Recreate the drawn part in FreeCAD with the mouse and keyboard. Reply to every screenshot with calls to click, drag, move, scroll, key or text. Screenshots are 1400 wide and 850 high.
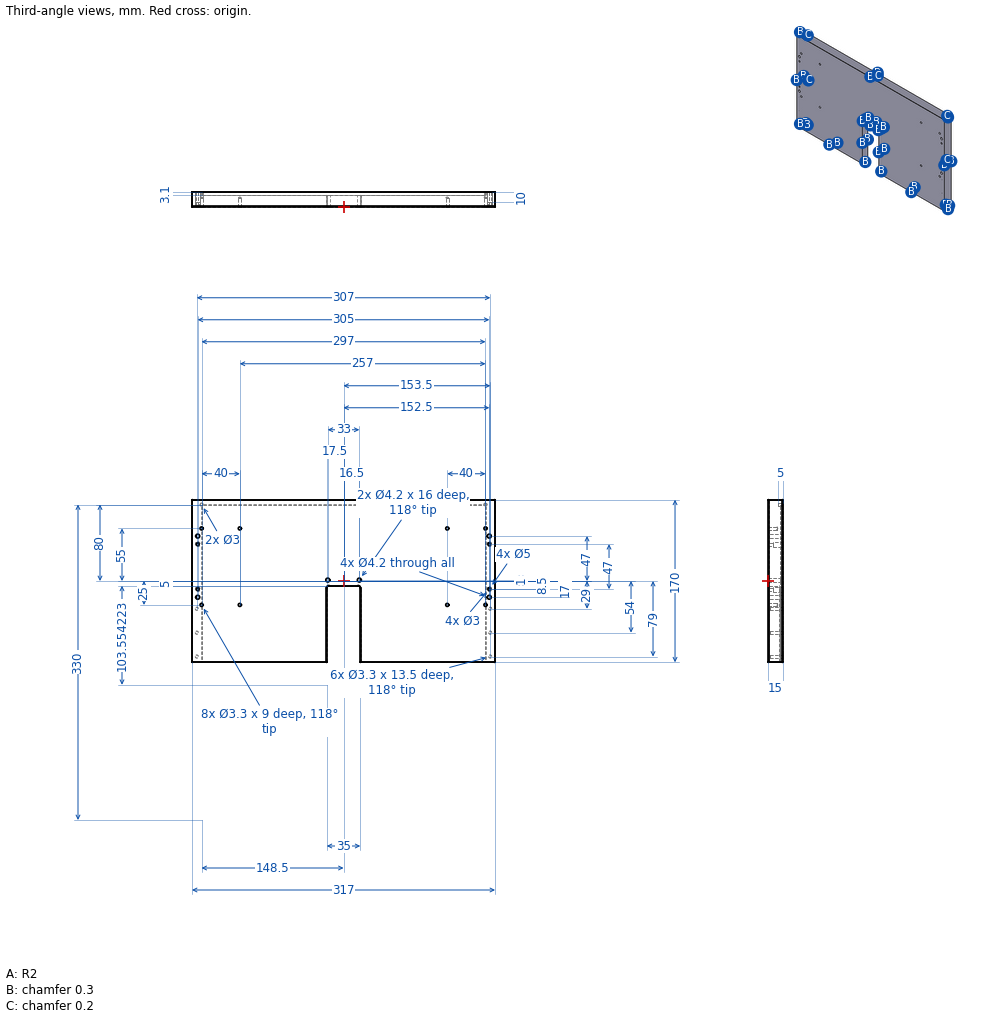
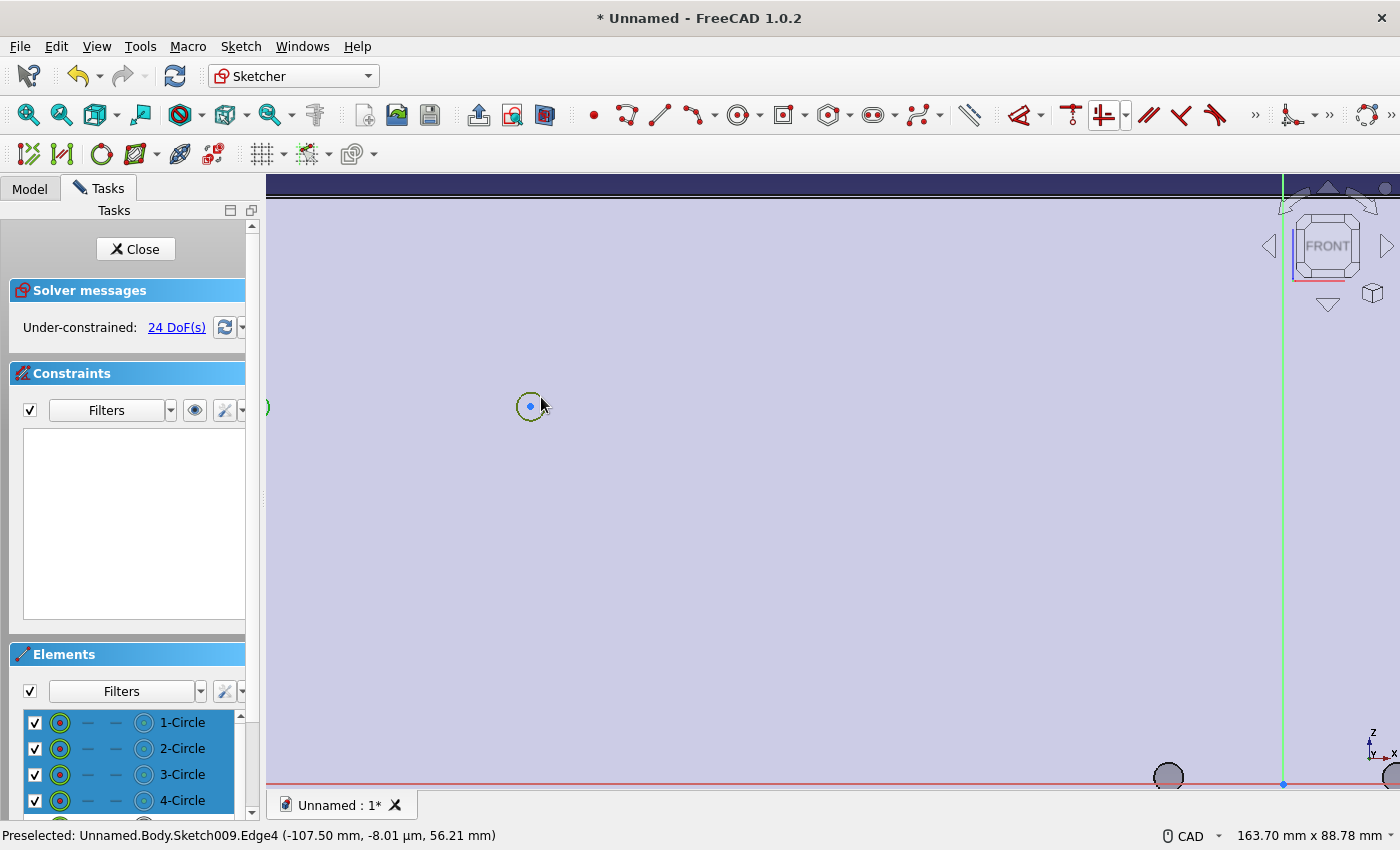
scroll(541, 396, down, 6)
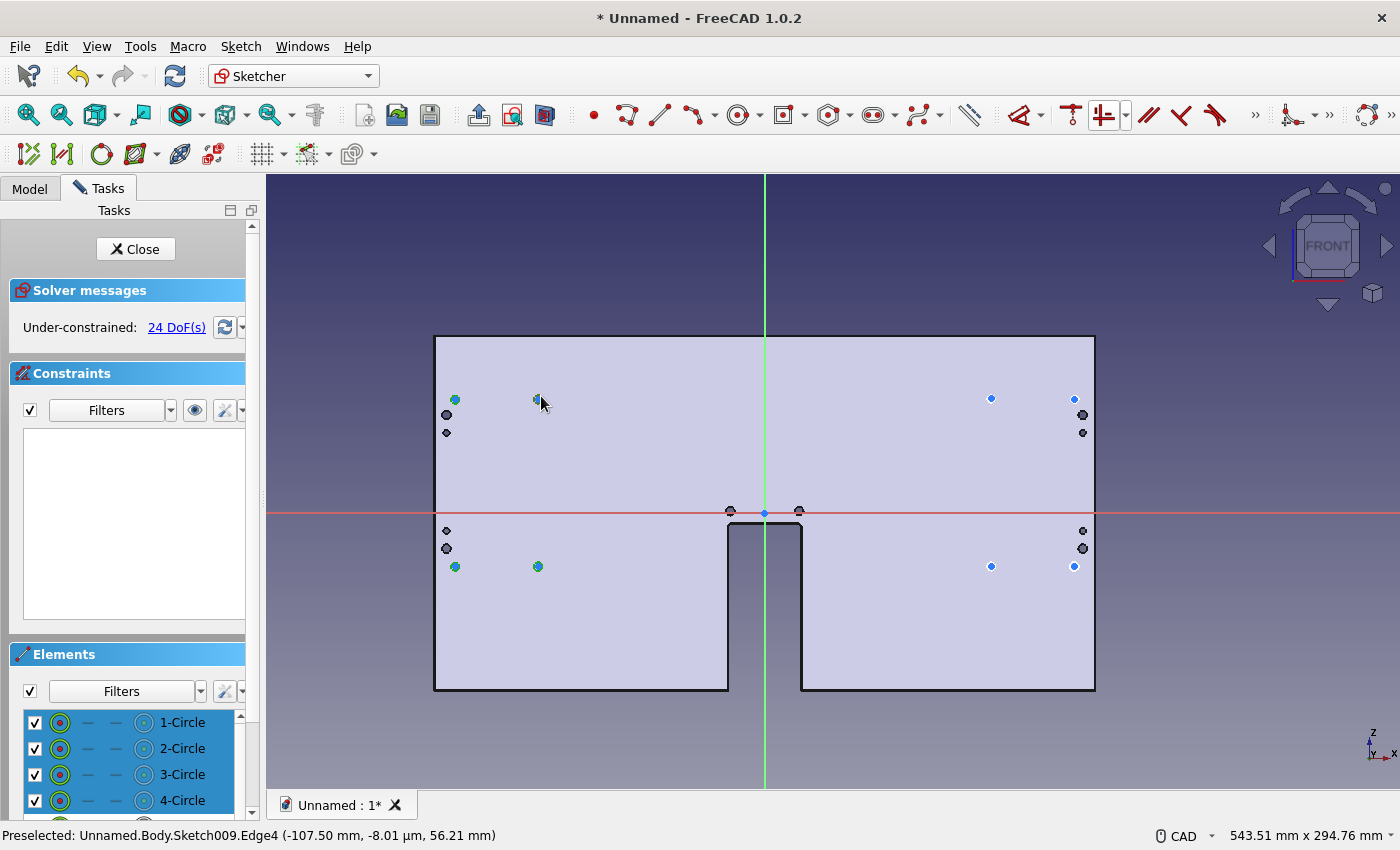
scroll(1077, 563, up, 6)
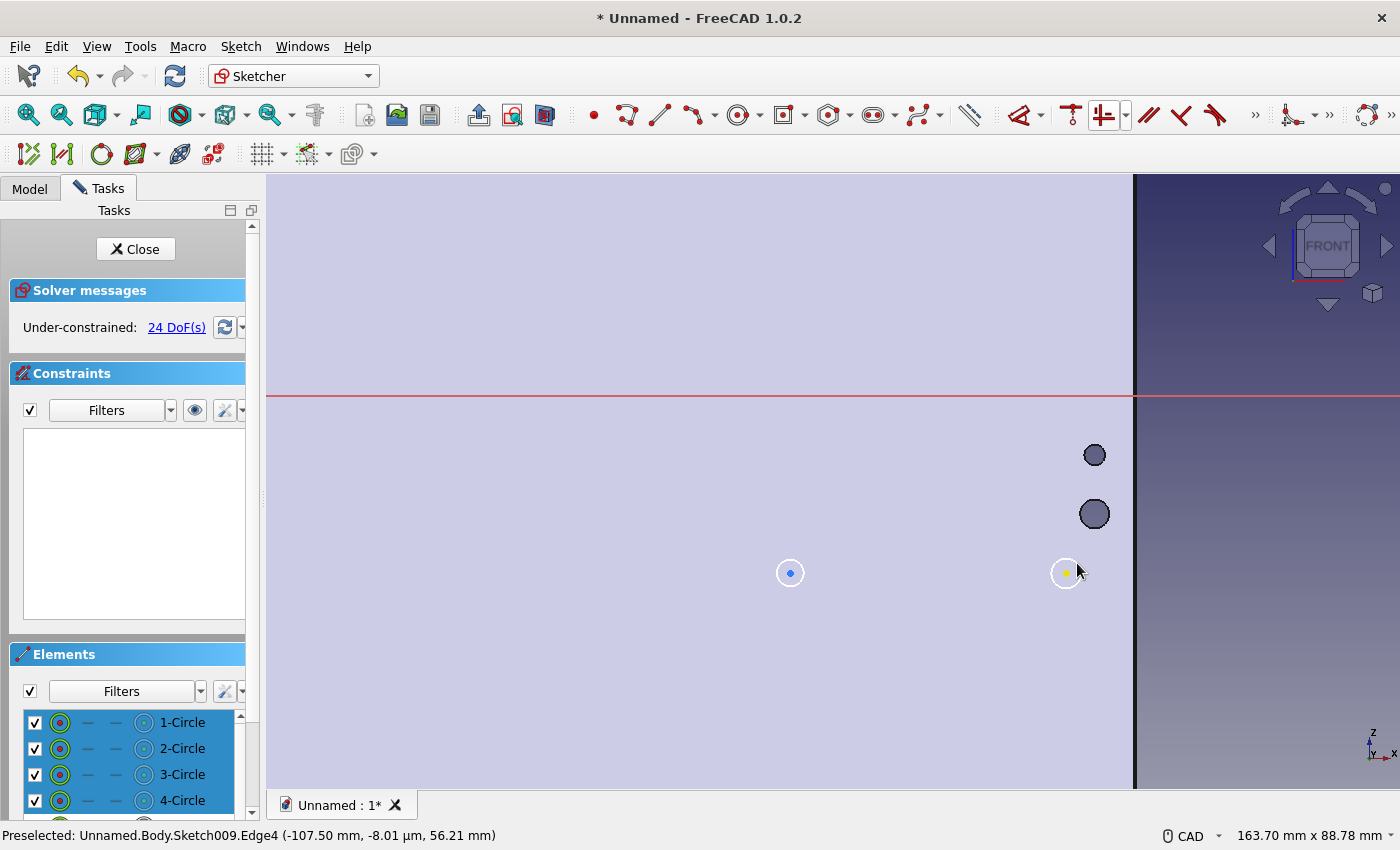
click(1077, 563)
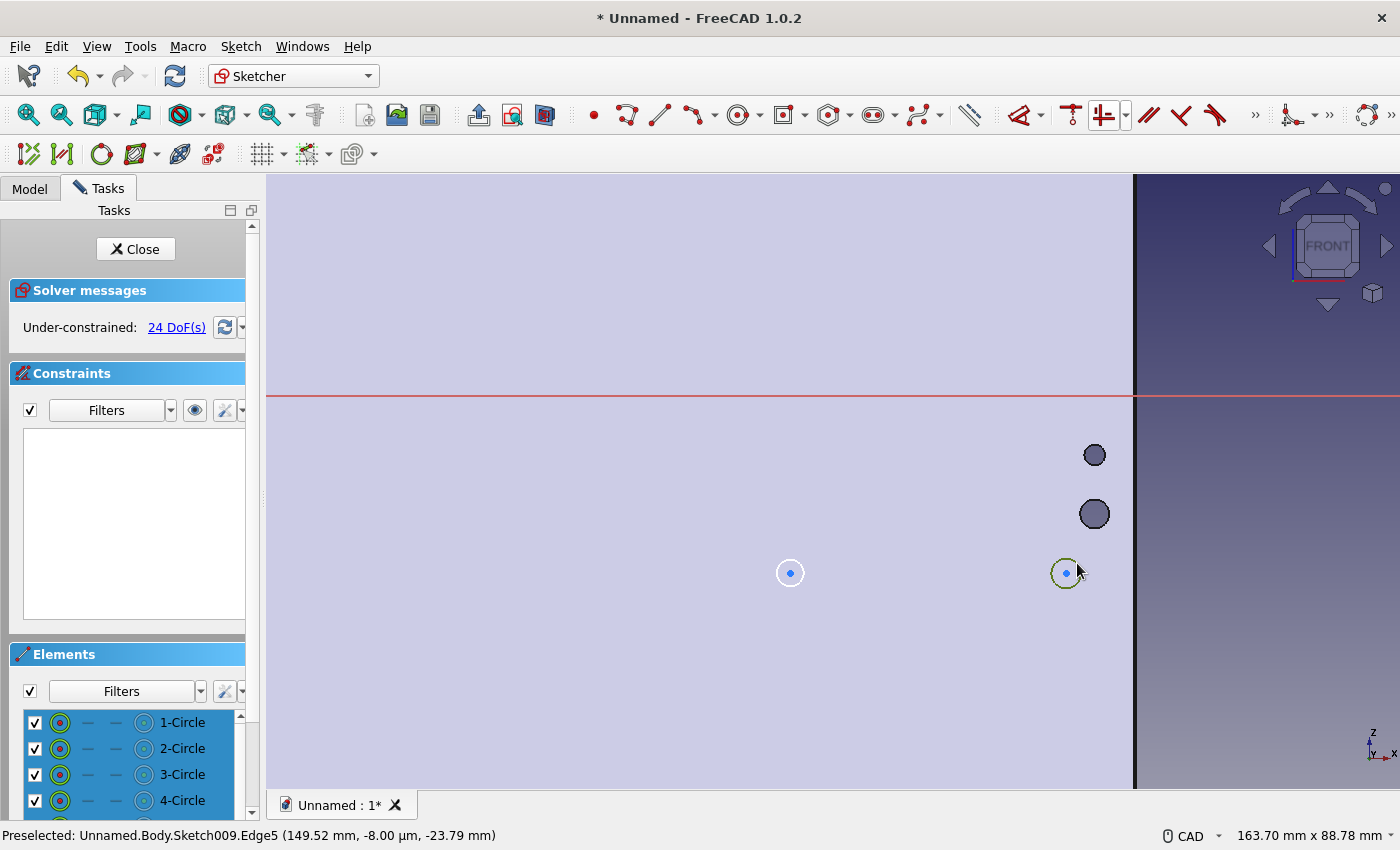
click(800, 564)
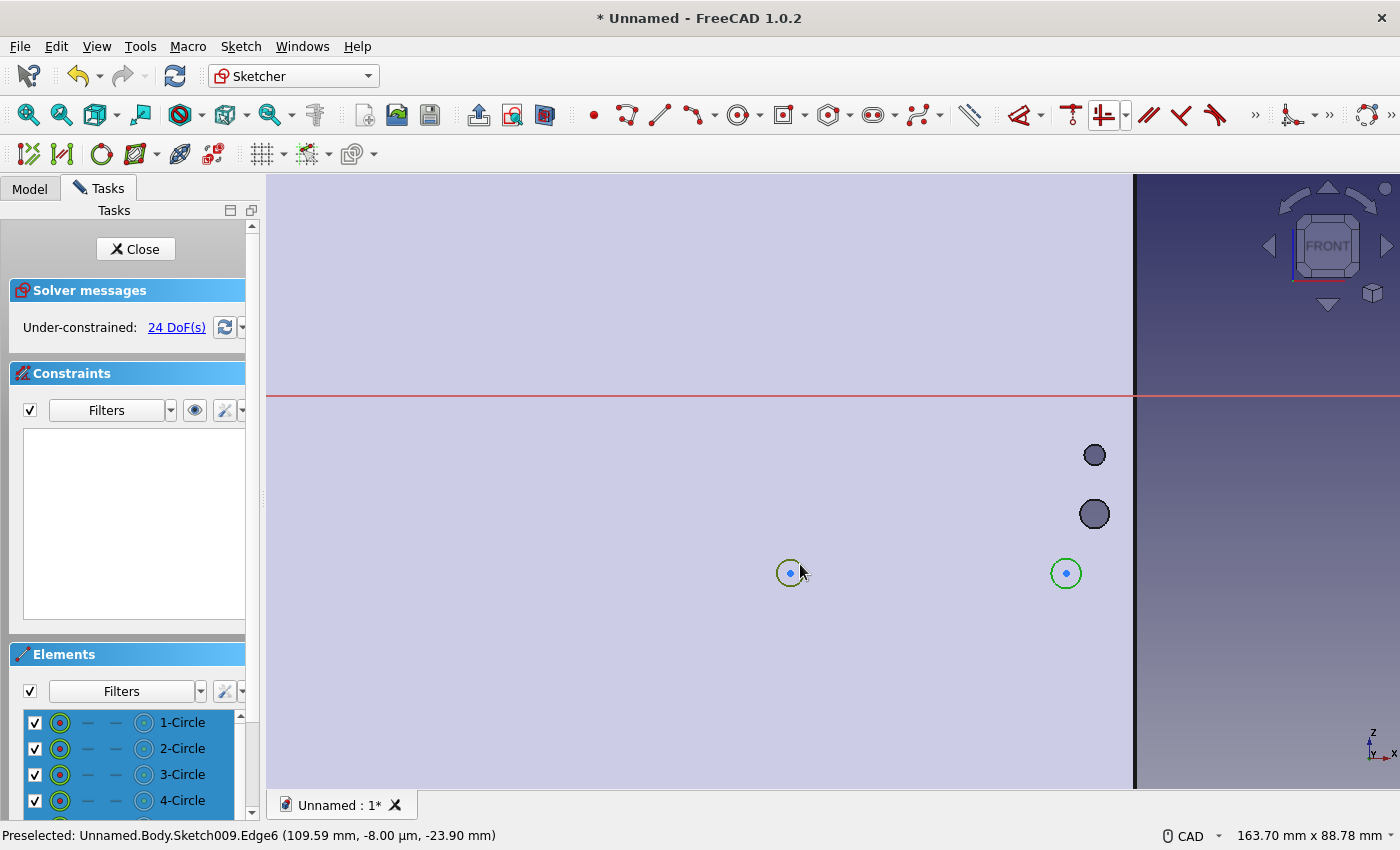
scroll(1077, 563, down, 6)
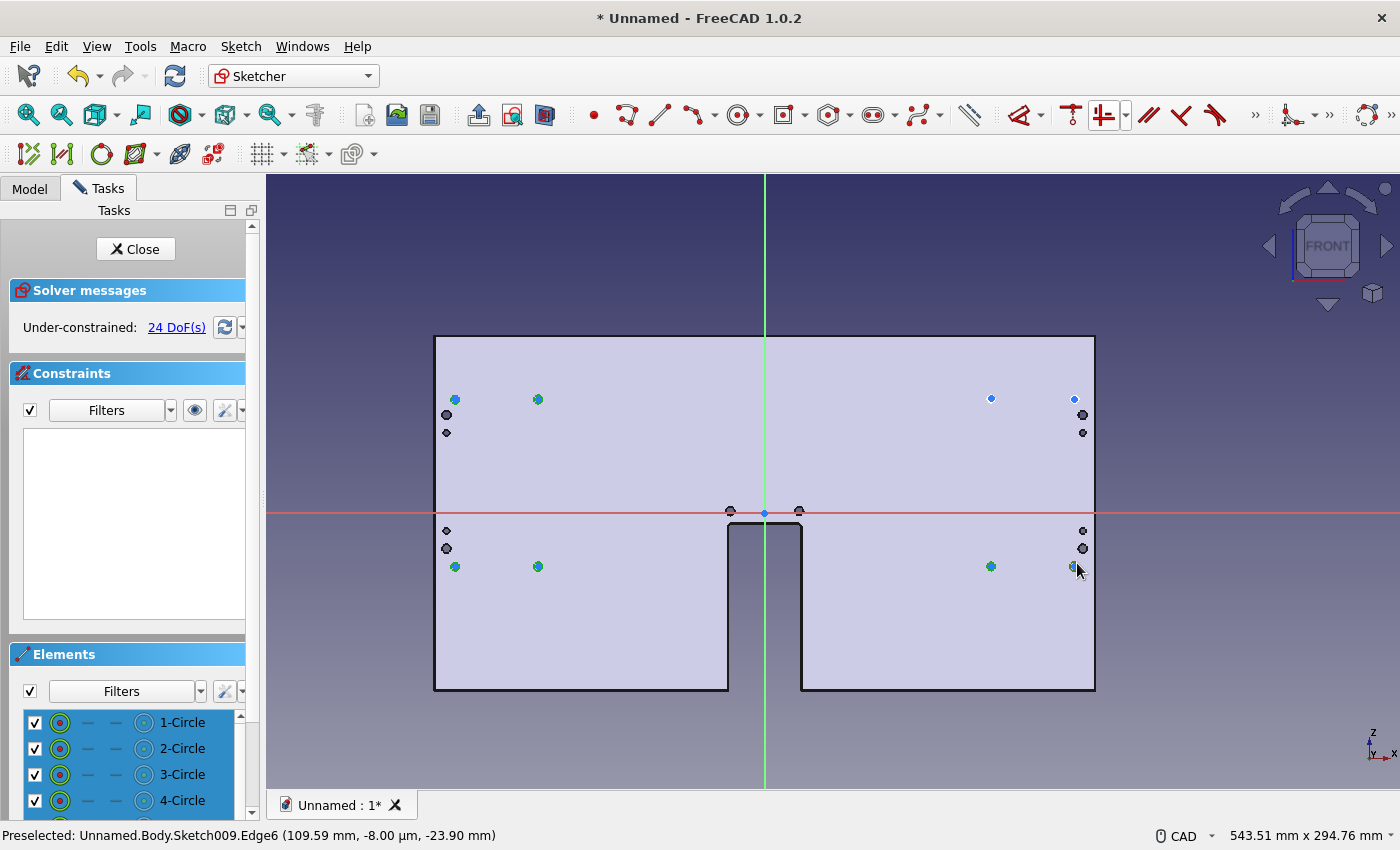
scroll(1078, 397, up, 7)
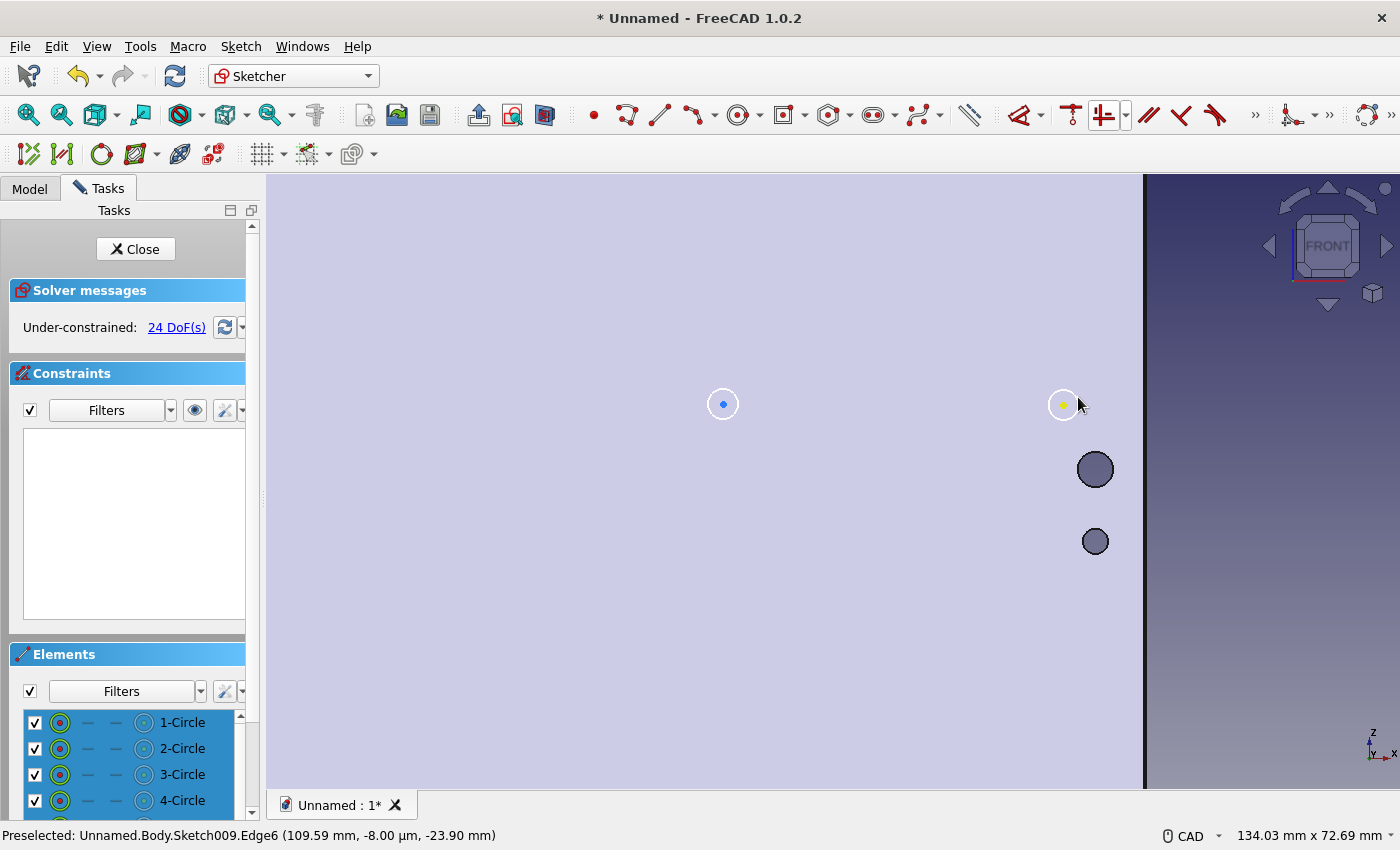
click(1074, 394)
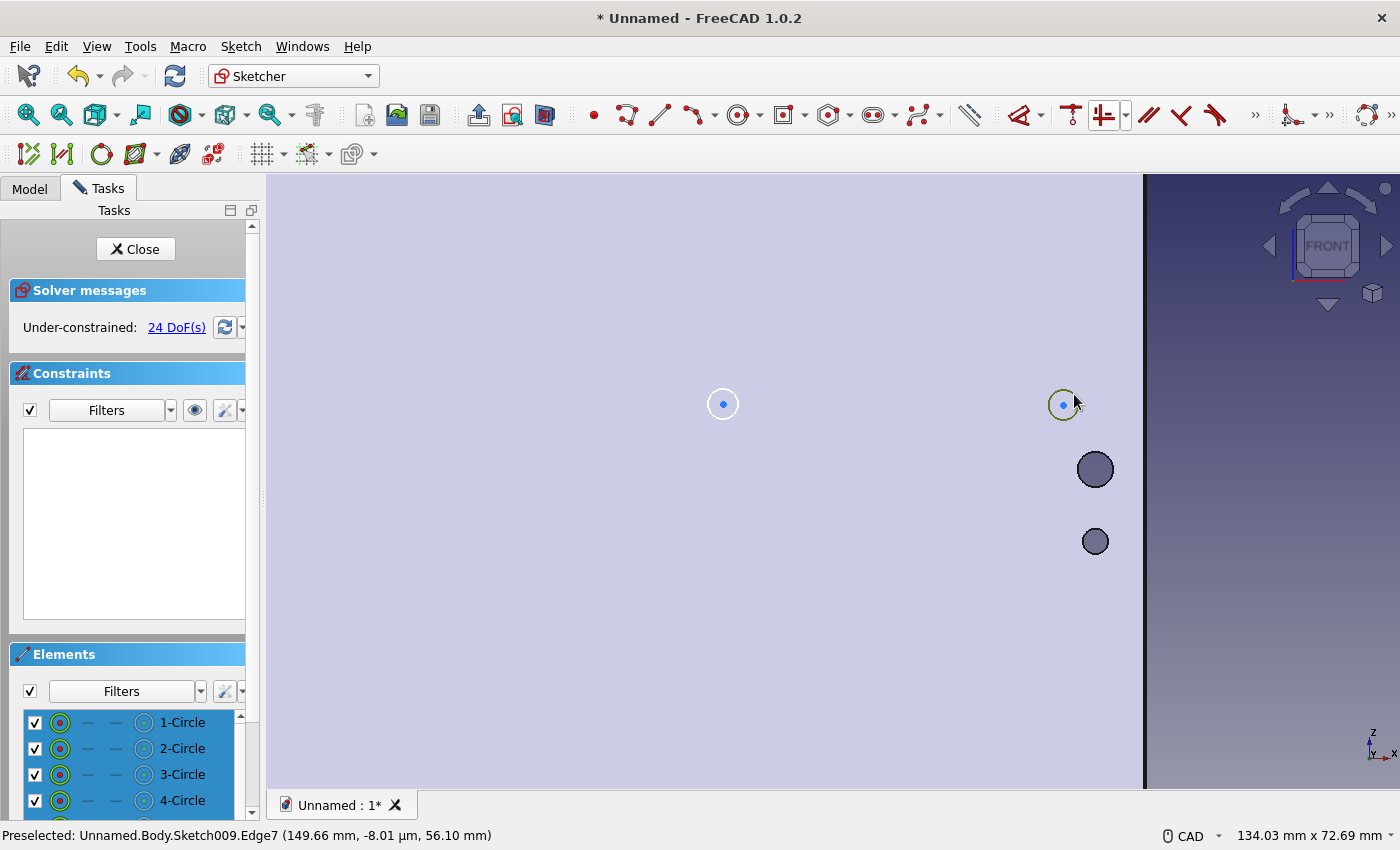
click(734, 393)